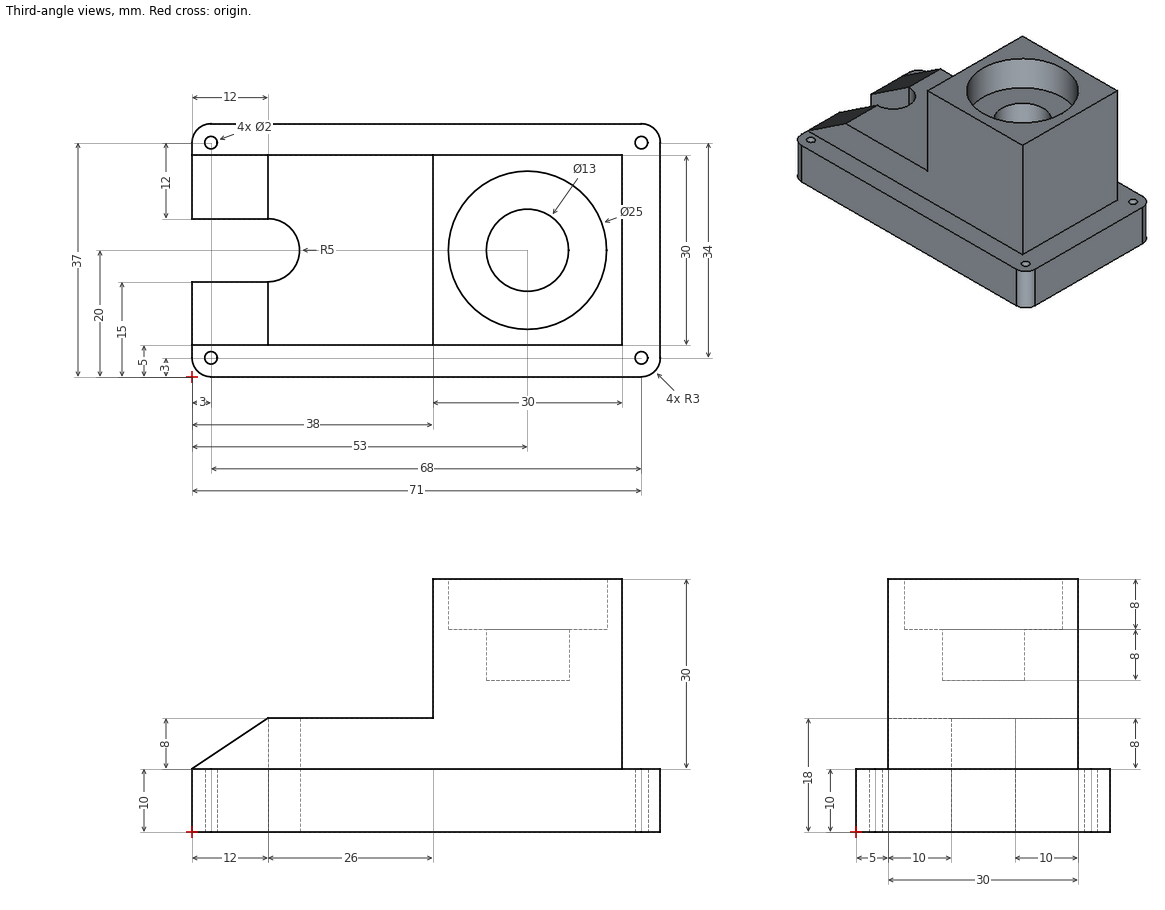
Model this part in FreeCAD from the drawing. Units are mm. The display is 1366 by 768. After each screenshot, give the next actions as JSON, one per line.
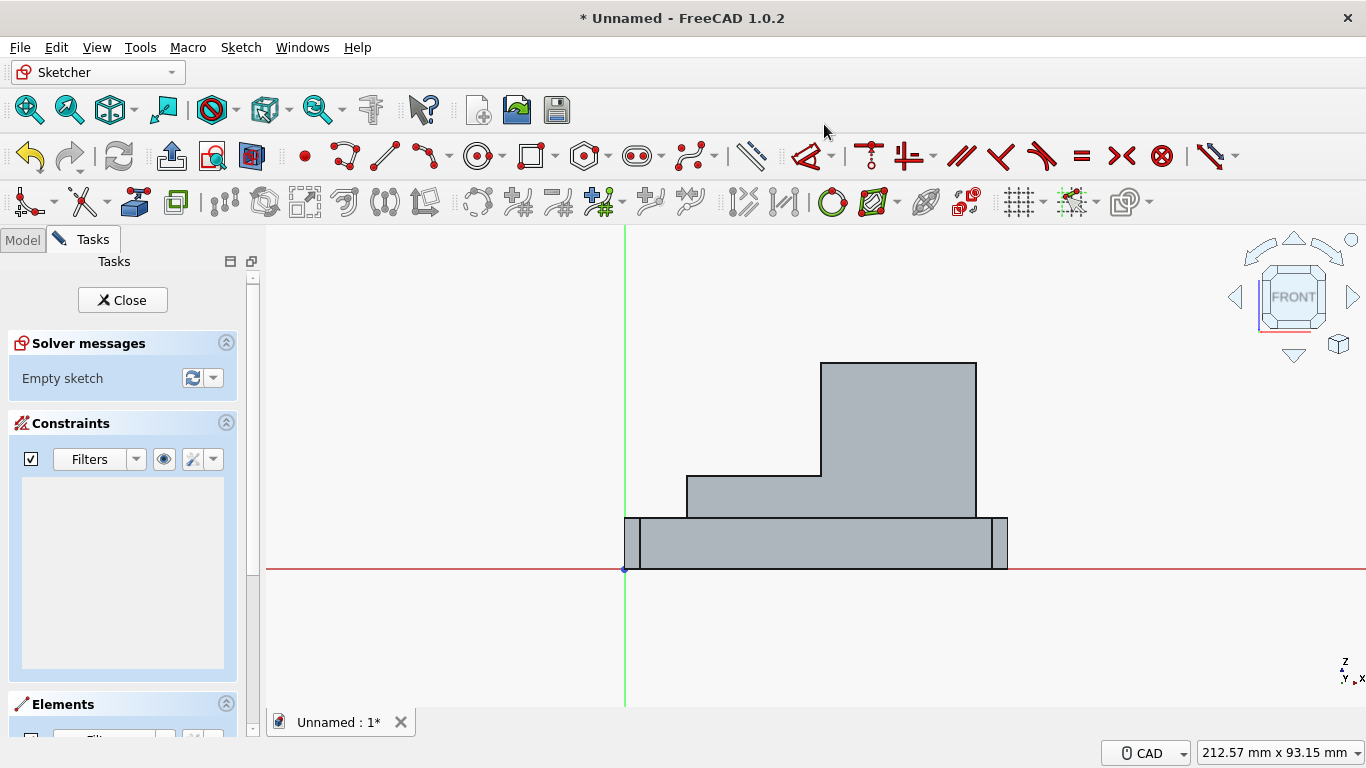
{"action": "scroll", "coordinate": [616, 547], "scroll_direction": "up", "scroll_amount": 6}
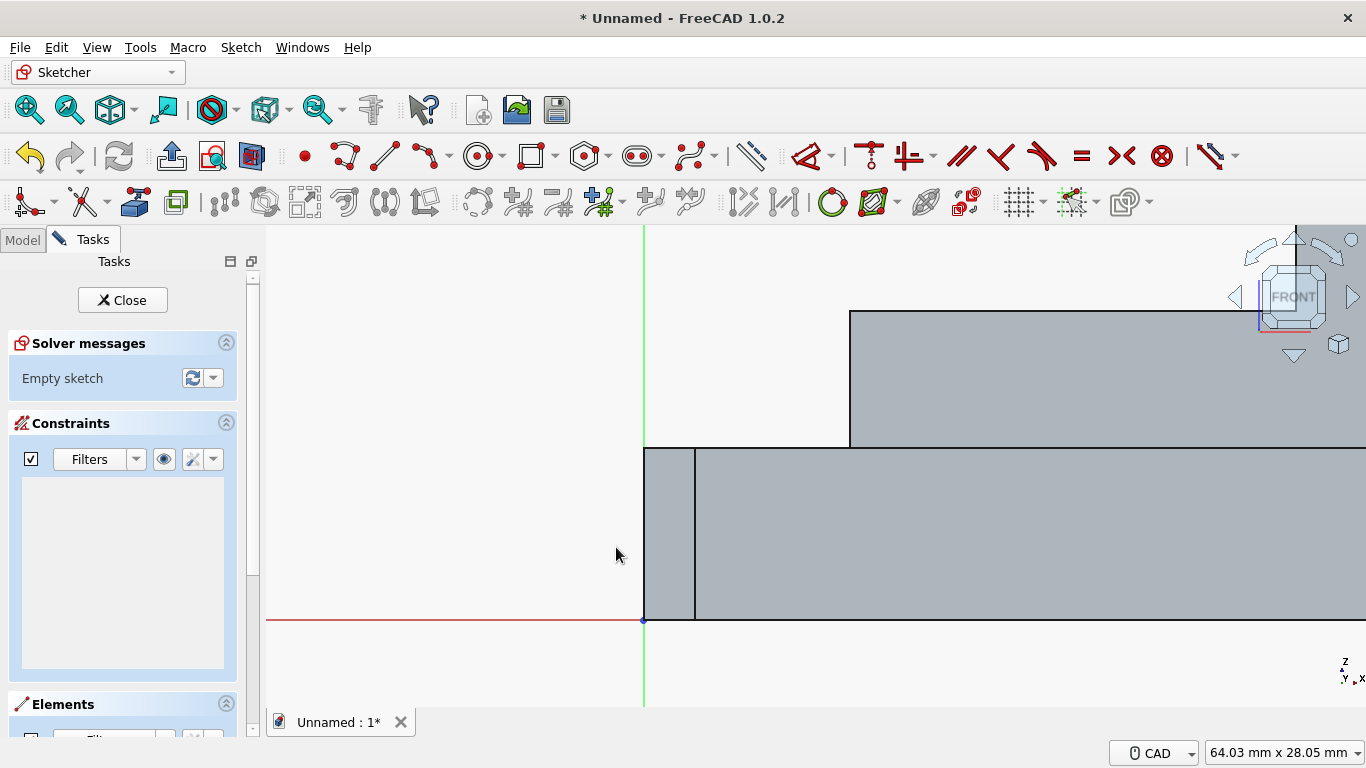
{"action": "left_click", "coordinate": [346, 156]}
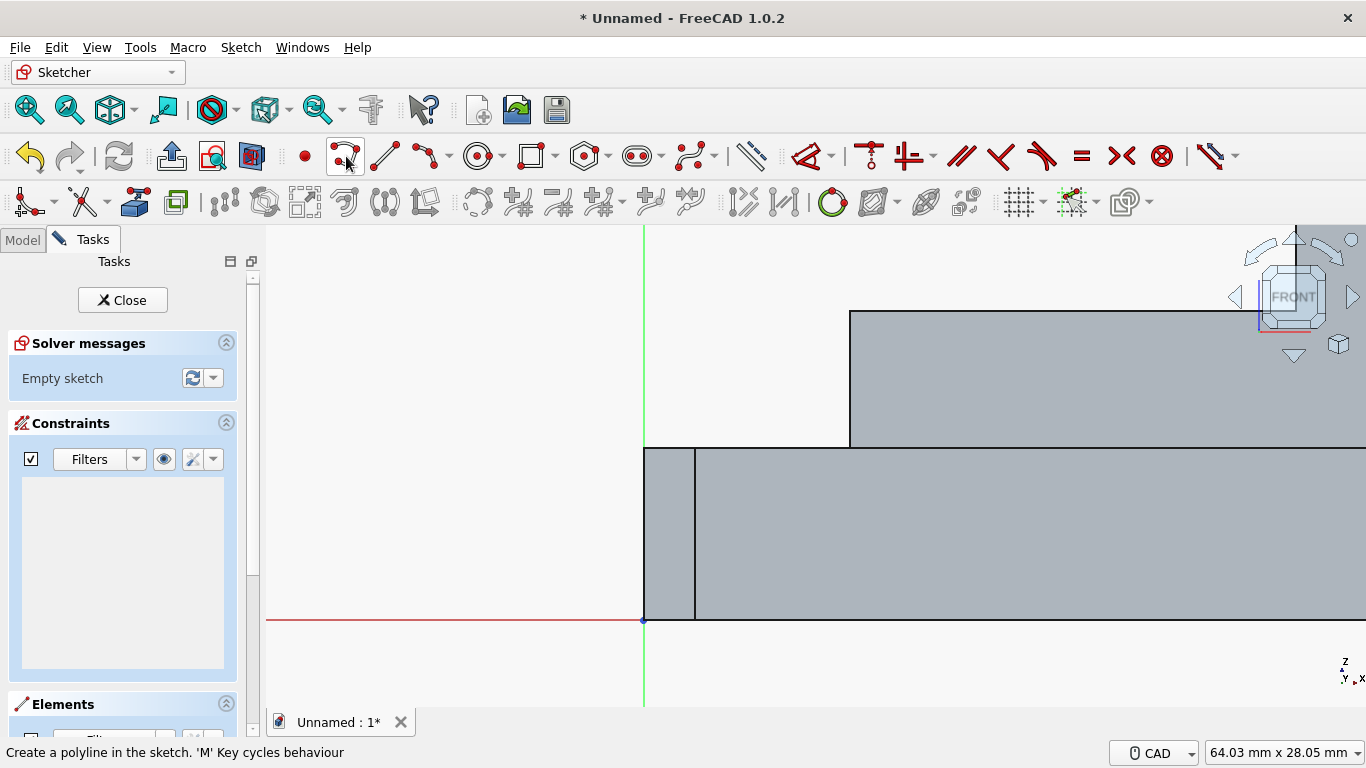
{"action": "left_click", "coordinate": [644, 448]}
{"action": "left_click", "coordinate": [850, 448]}
{"action": "left_click", "coordinate": [850, 311]}
{"action": "left_click", "coordinate": [644, 449]}
{"action": "key", "text": "Escape"}
{"action": "key", "text": "Escape"}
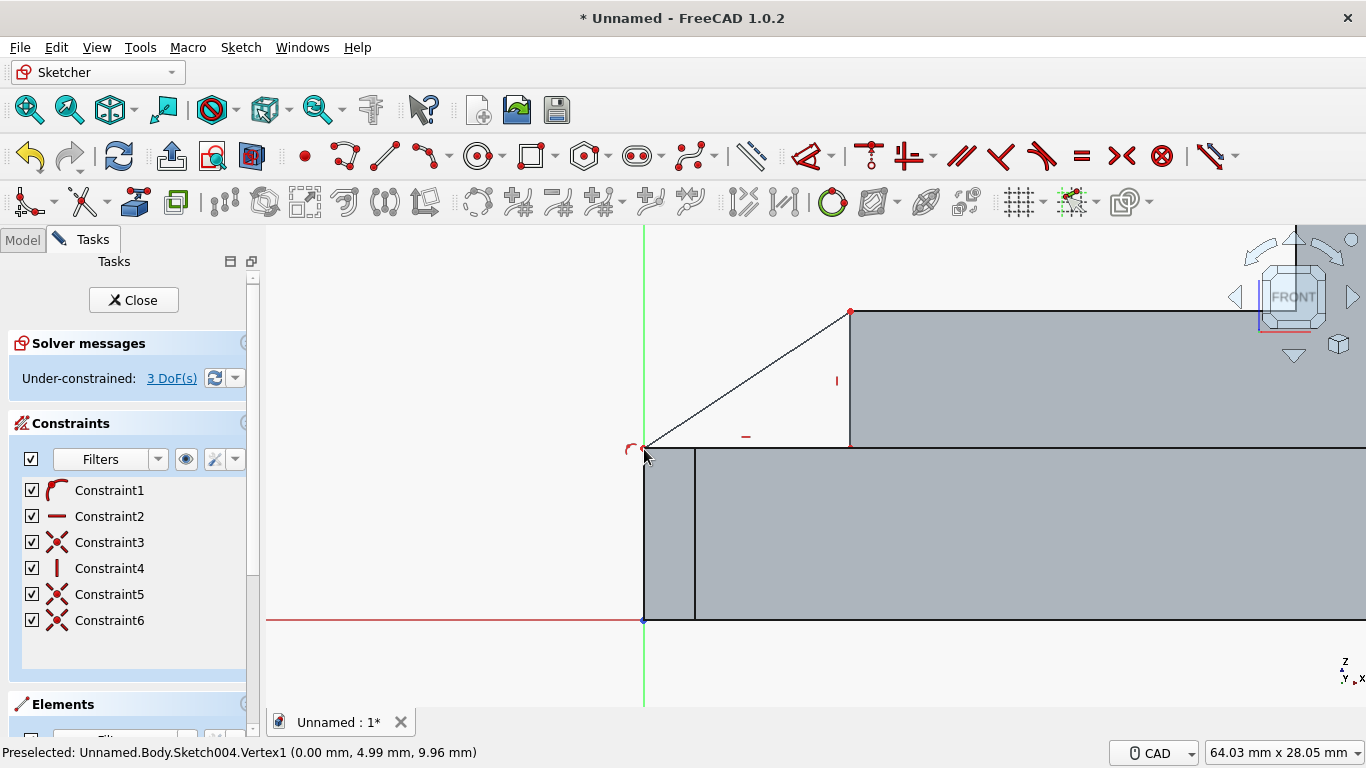
{"action": "left_click", "coordinate": [806, 156]}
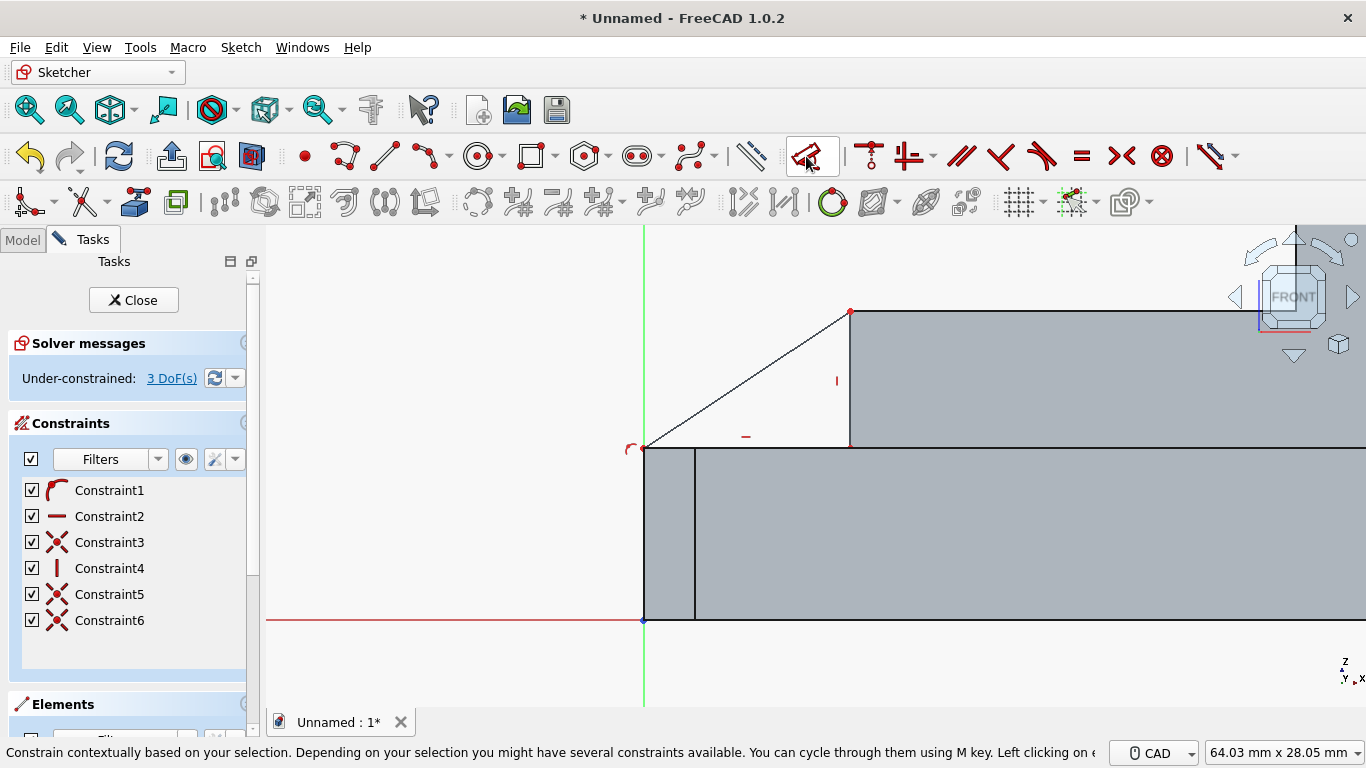
{"action": "left_click", "coordinate": [850, 408]}
{"action": "left_click", "coordinate": [884, 380]}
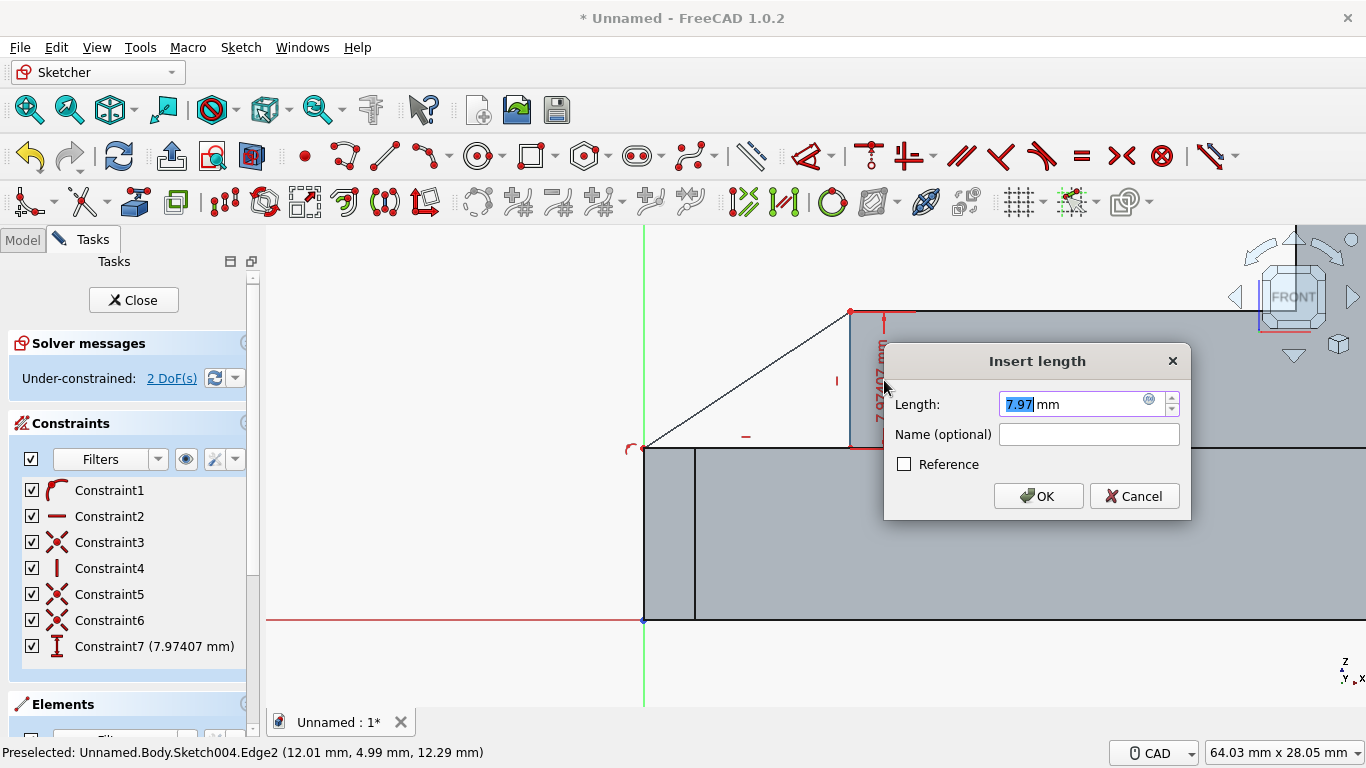
{"action": "type", "text": "8"}
{"action": "key", "text": "Return"}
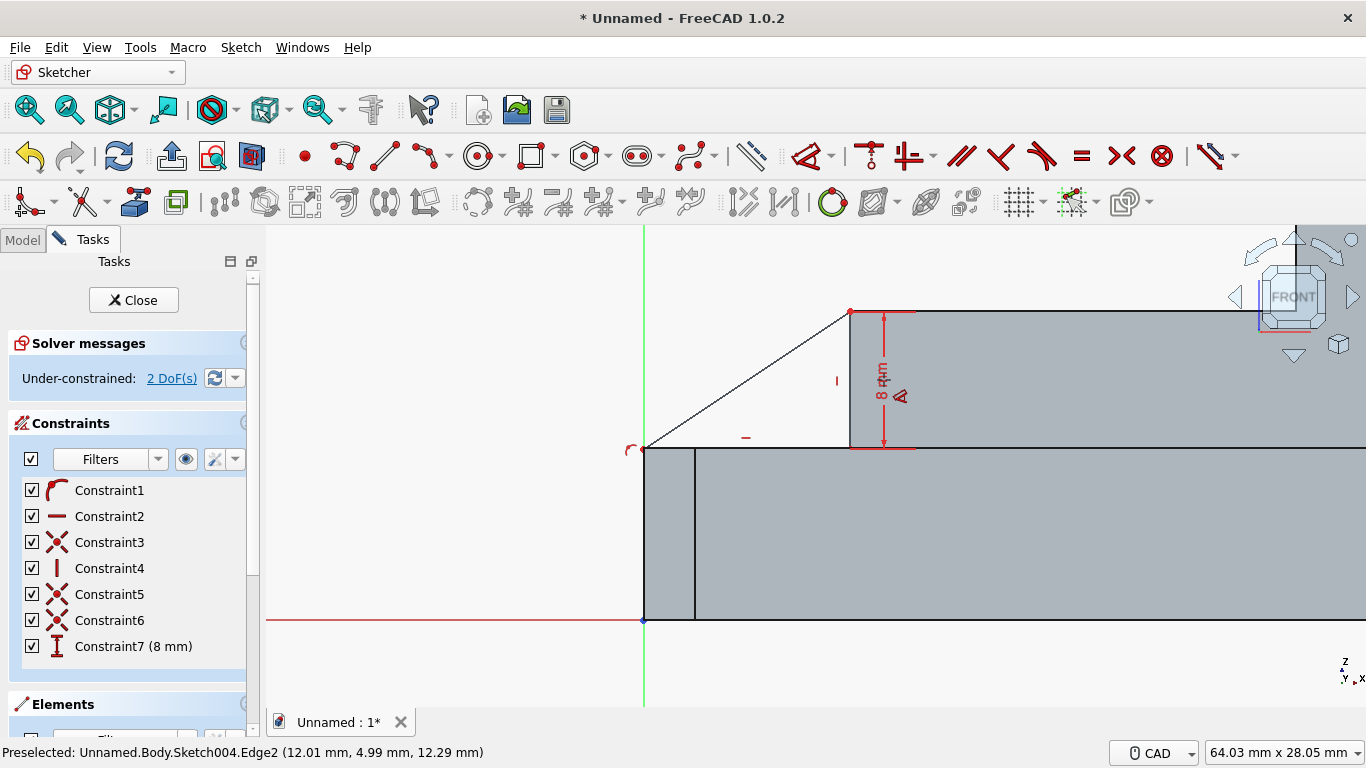
{"action": "left_click", "coordinate": [706, 449]}
{"action": "left_click", "coordinate": [747, 415]}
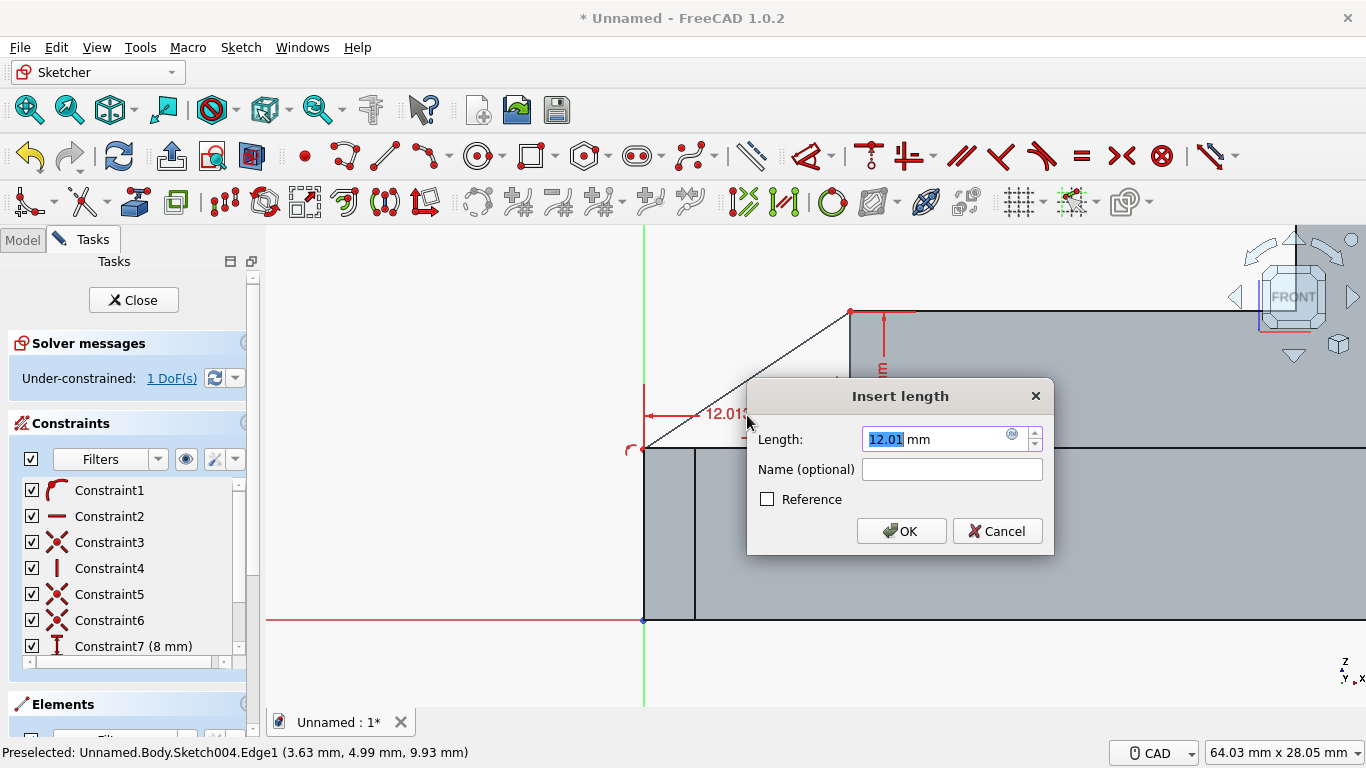
{"action": "type", "text": "12"}
{"action": "key", "text": "Return"}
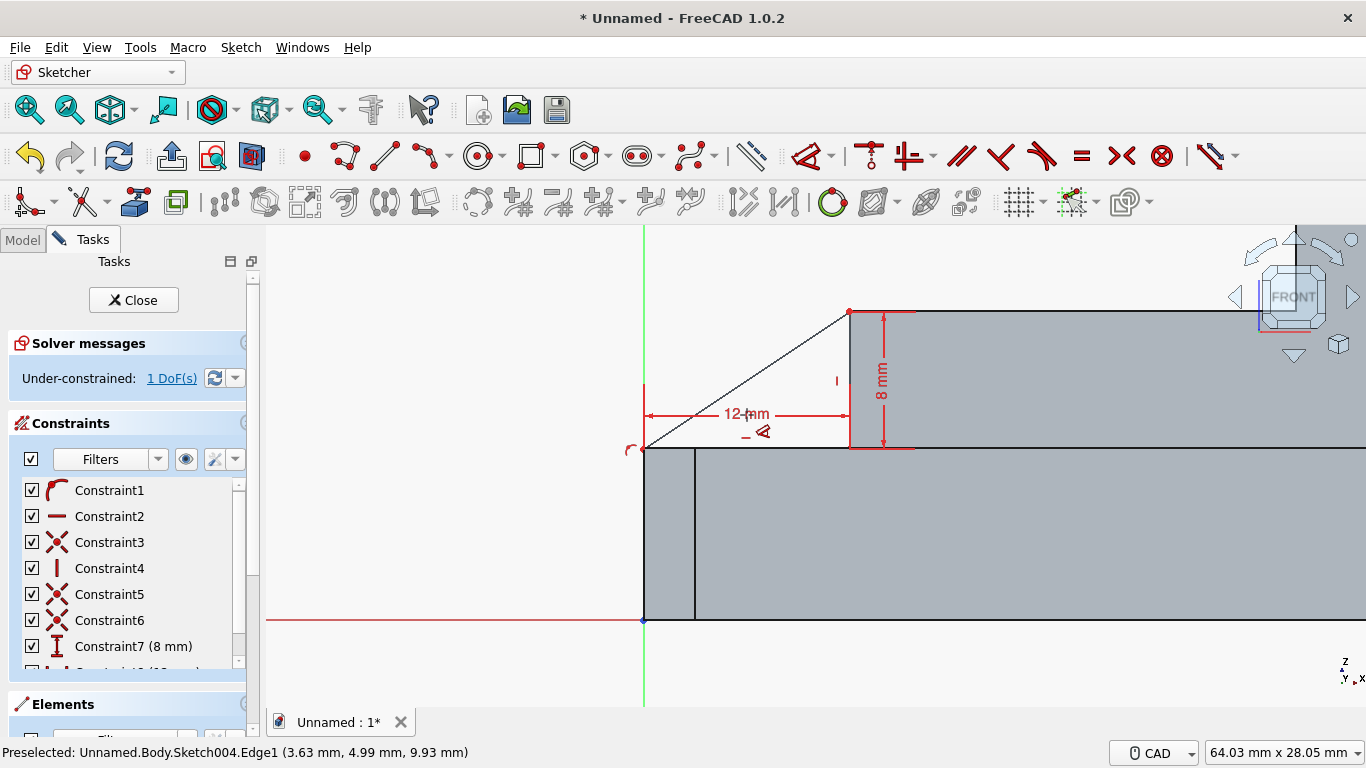
{"action": "left_click", "coordinate": [644, 449]}
{"action": "left_click", "coordinate": [610, 535]}